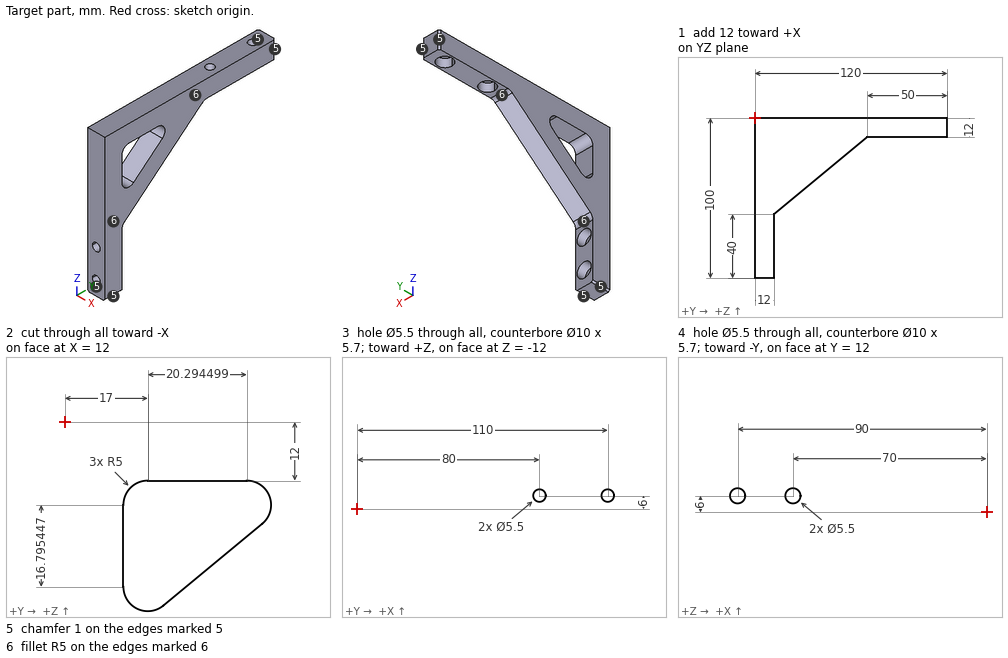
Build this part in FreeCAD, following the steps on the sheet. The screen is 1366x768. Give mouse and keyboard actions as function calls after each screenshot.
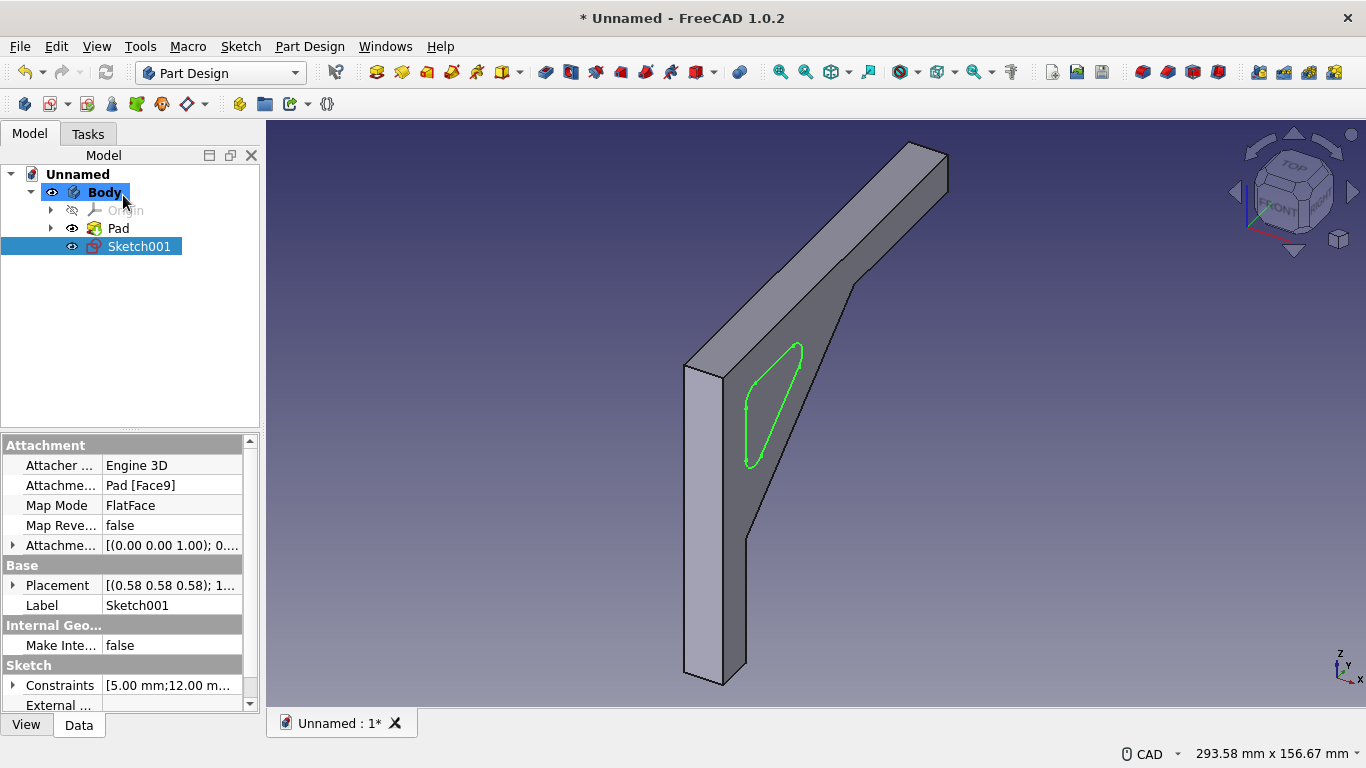
click(546, 72)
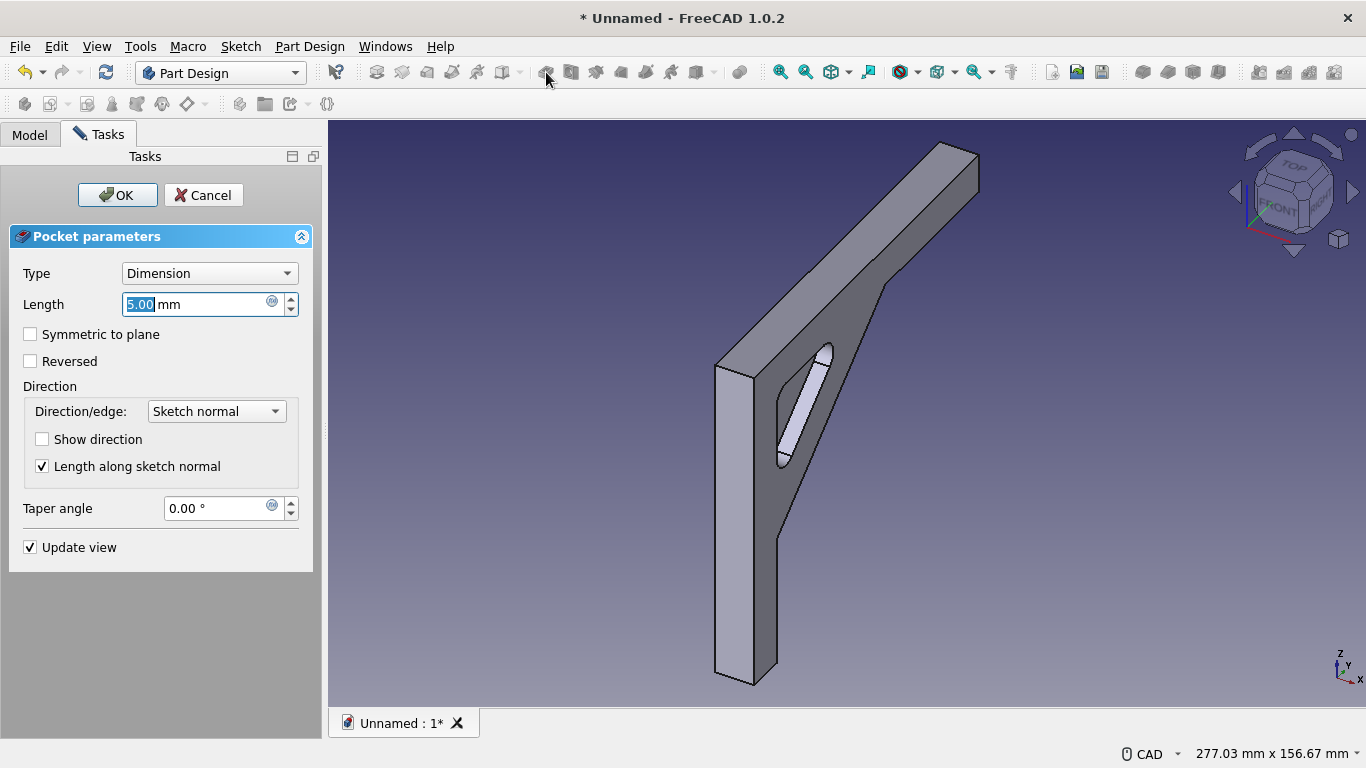
click(210, 274)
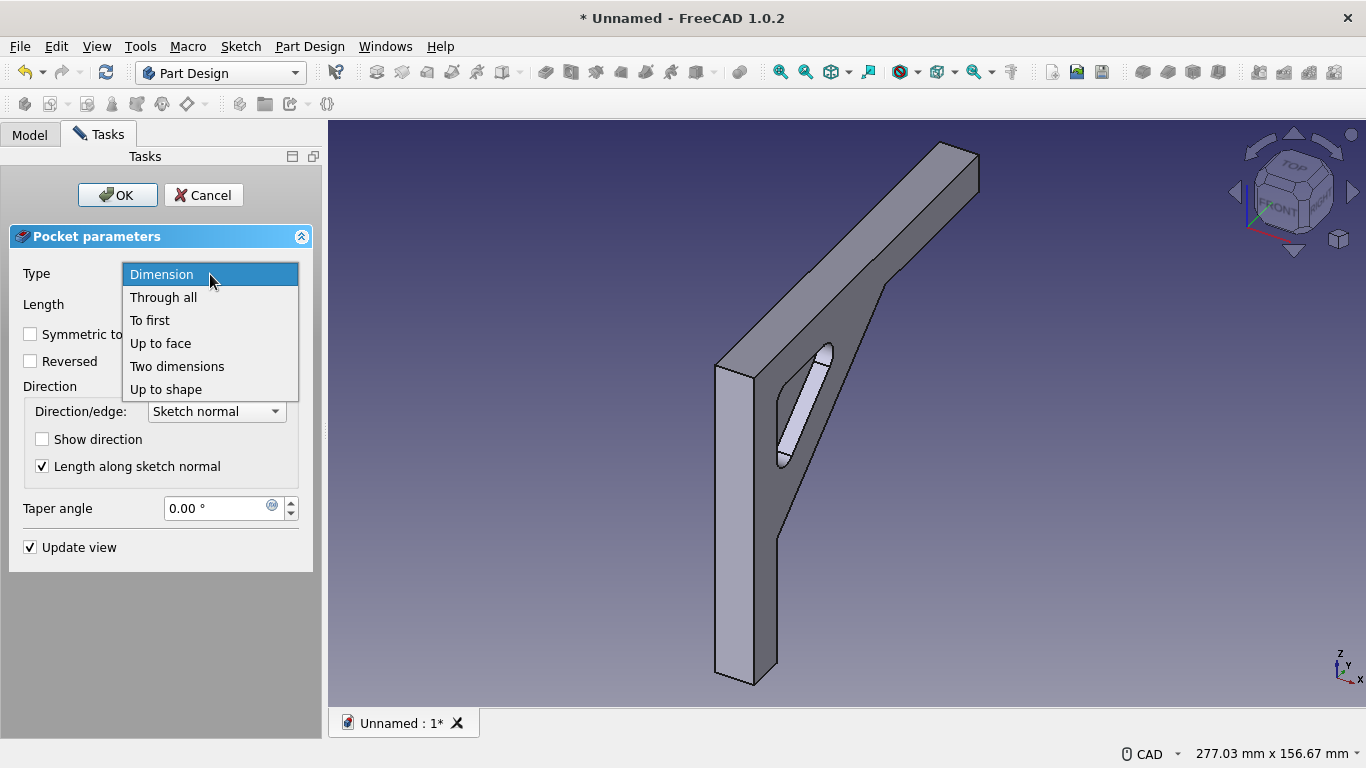
click(208, 298)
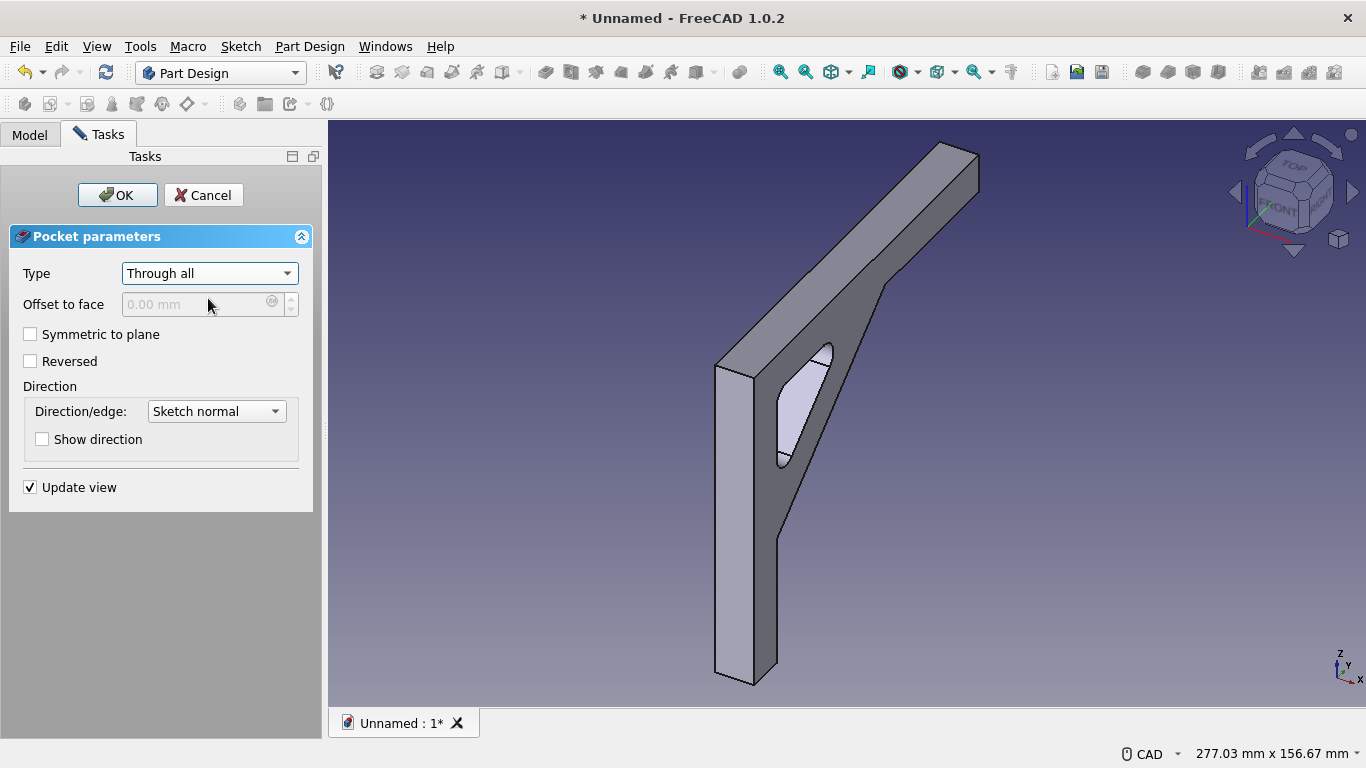
click(118, 195)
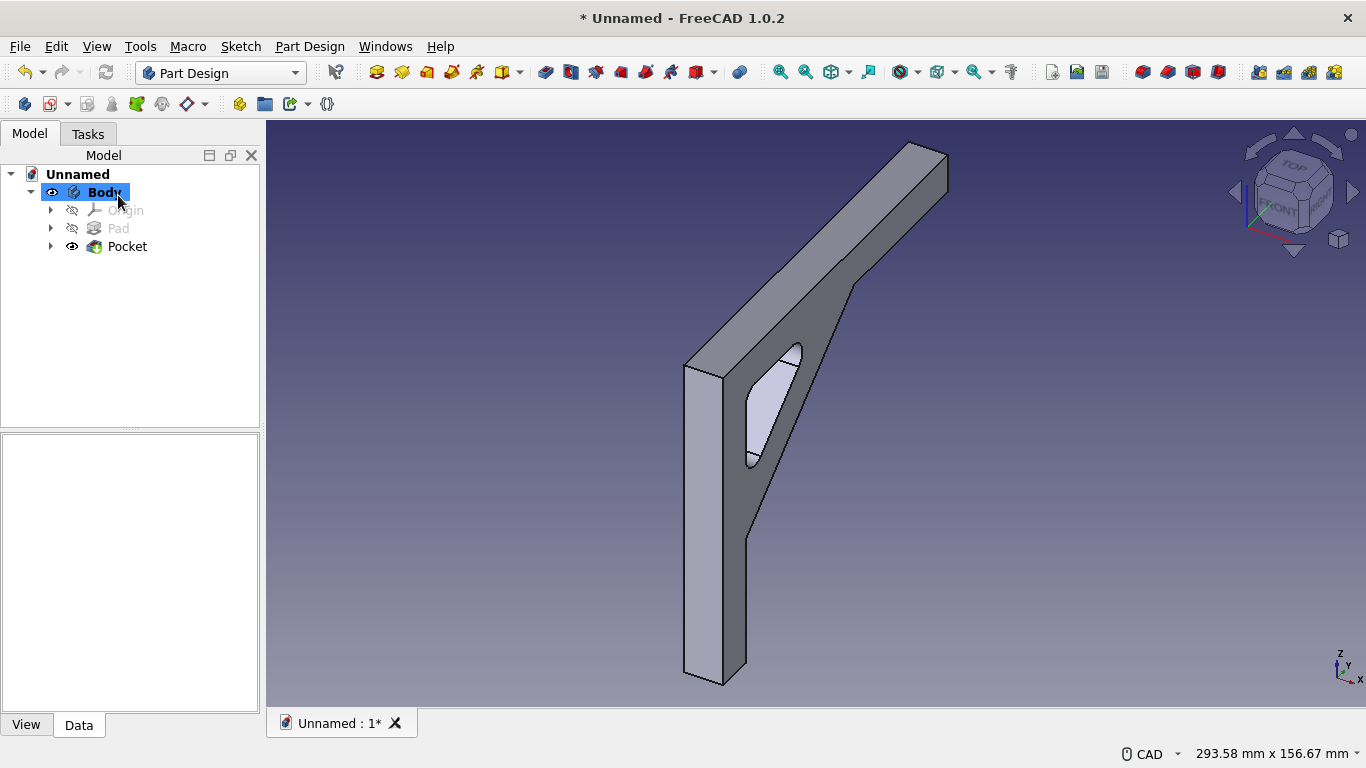
key(5)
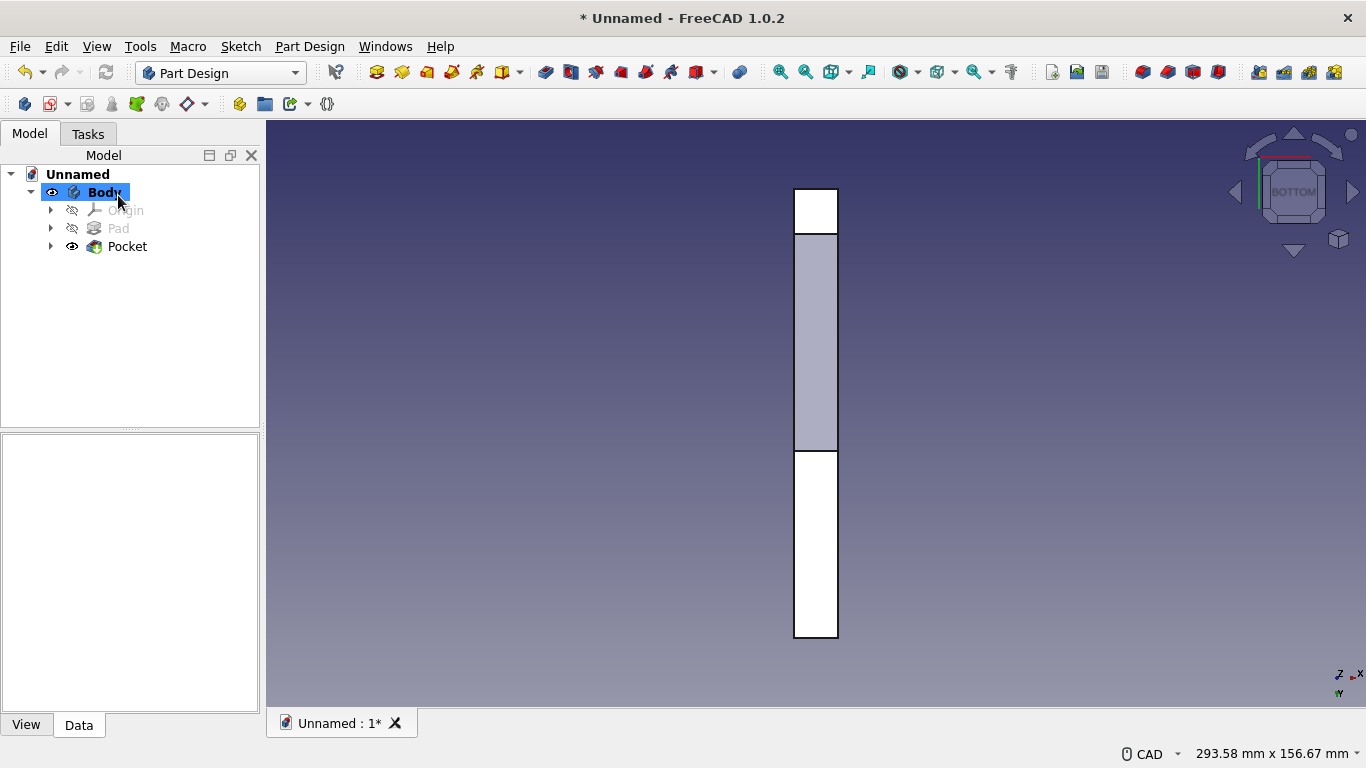
click(816, 597)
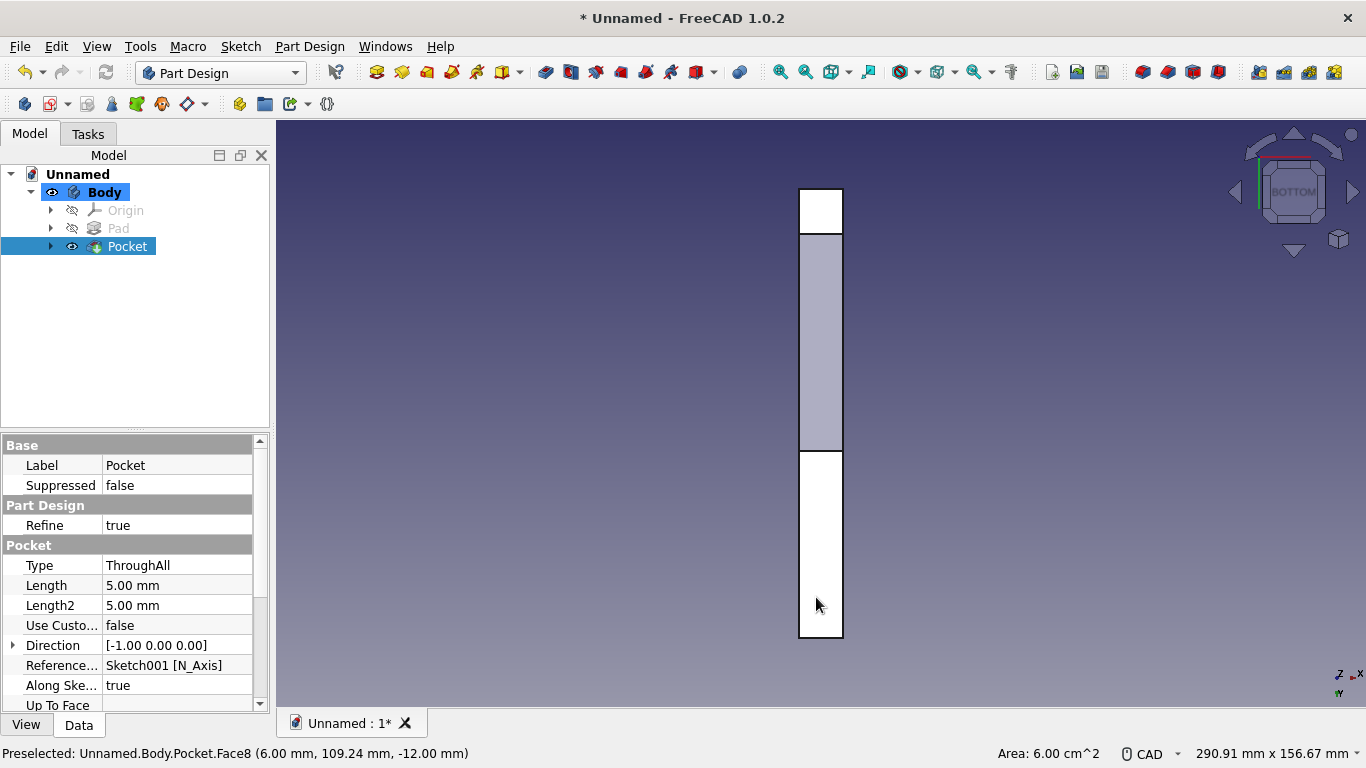
click(50, 104)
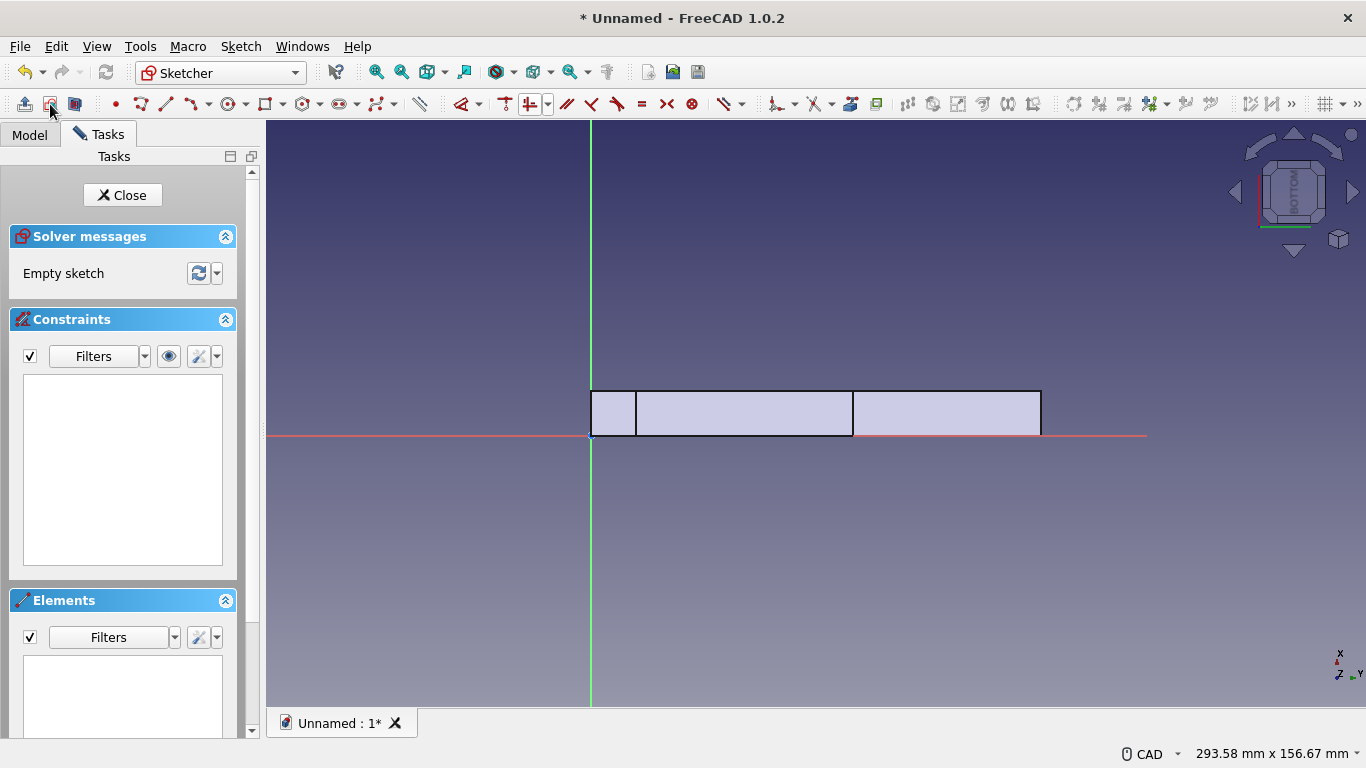
scroll(998, 413, up, 8)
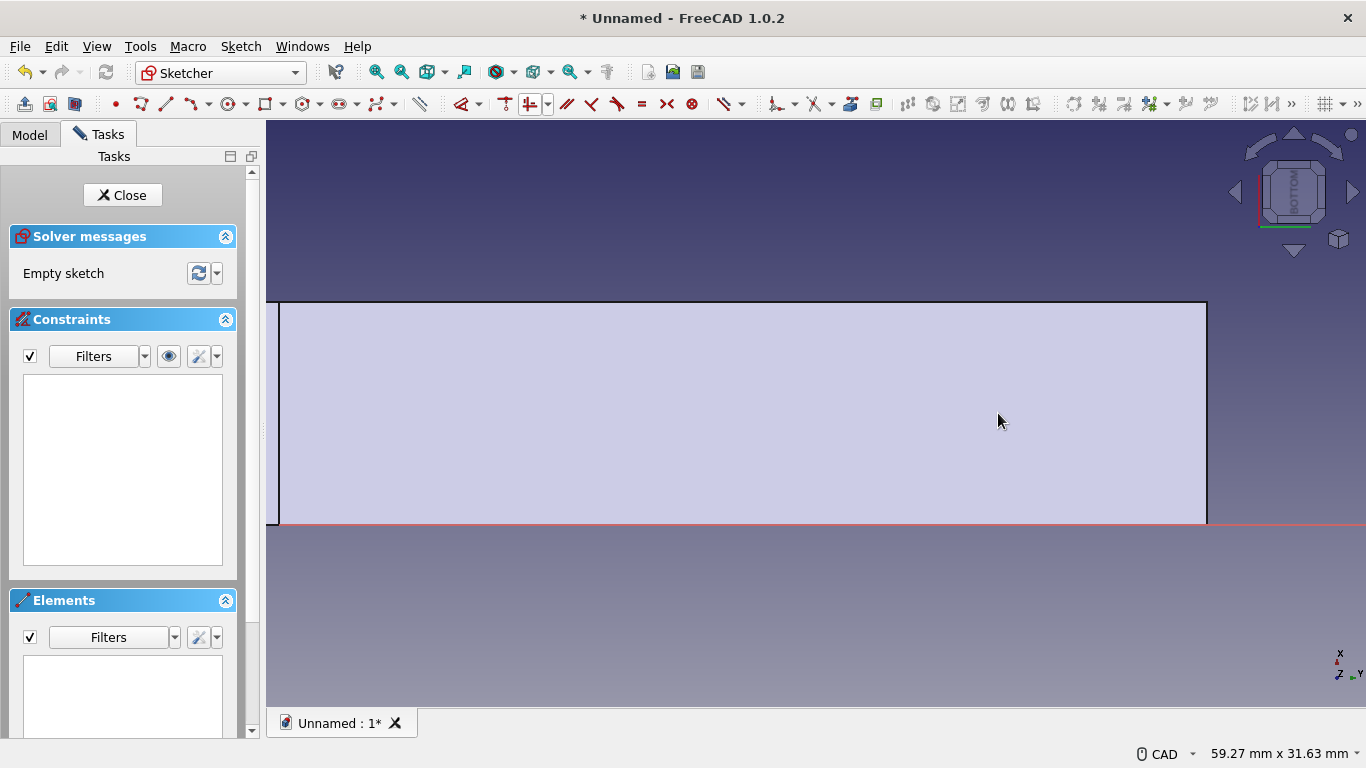
click(228, 104)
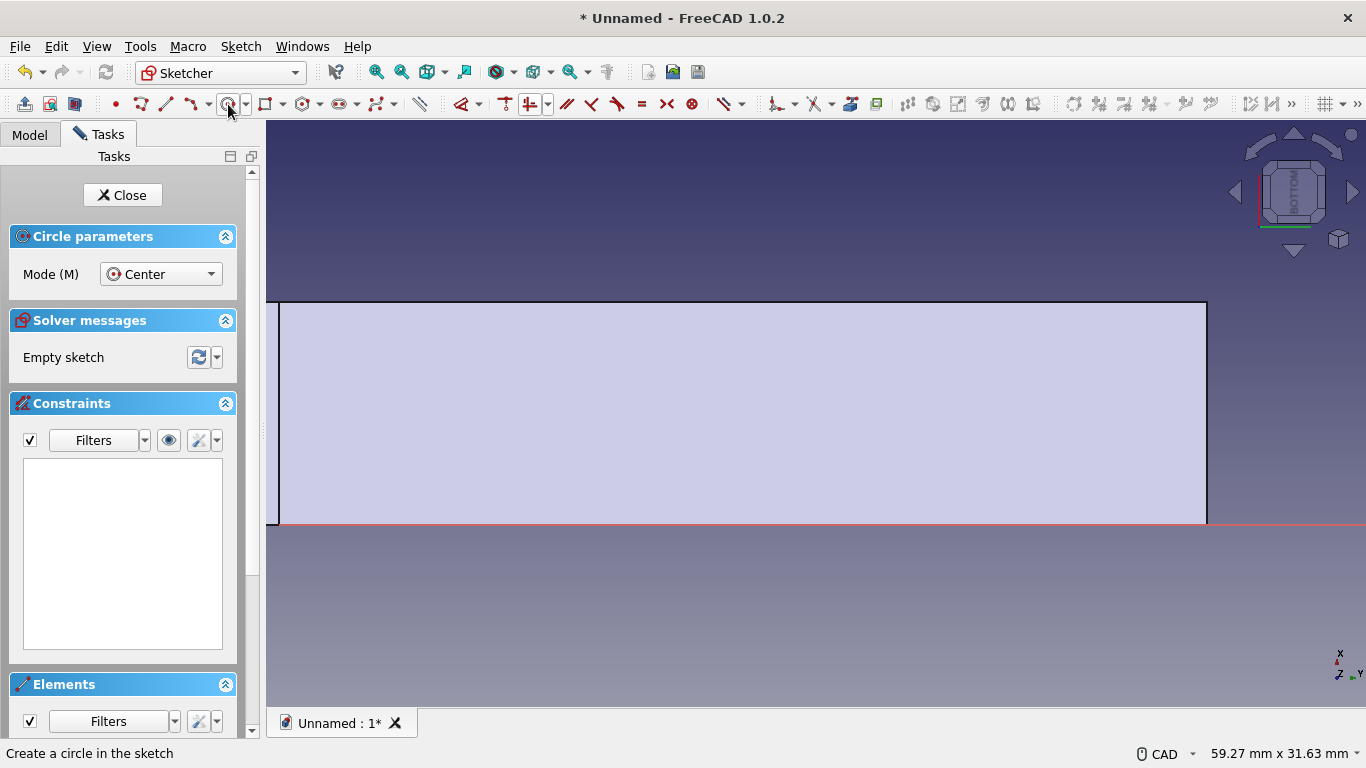
click(465, 413)
click(501, 377)